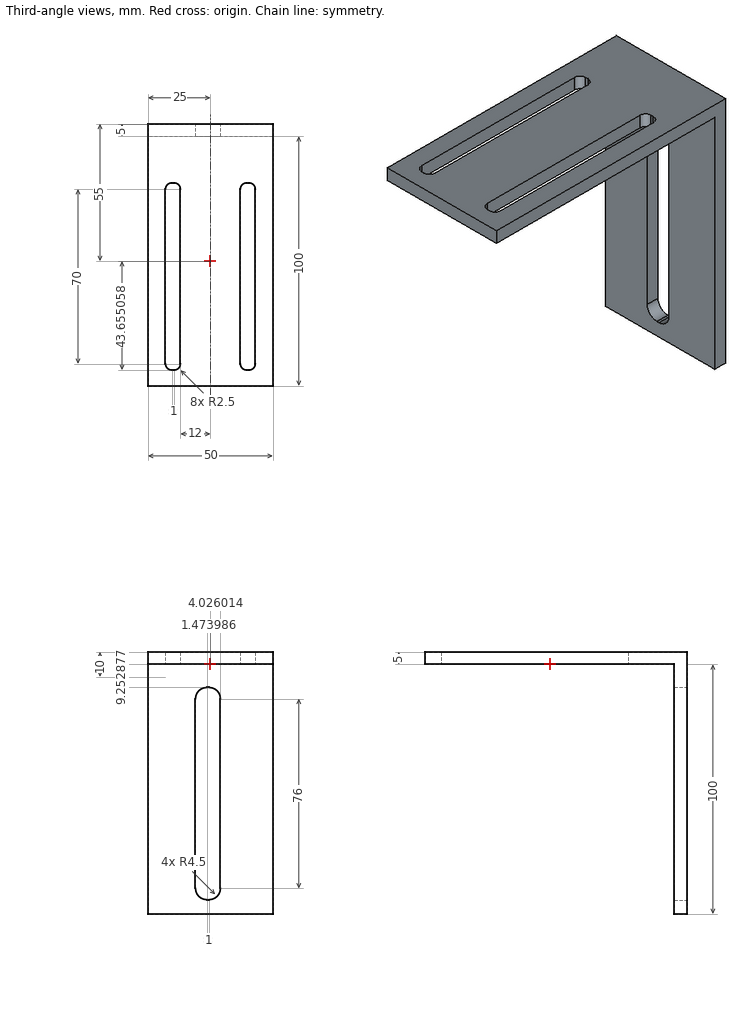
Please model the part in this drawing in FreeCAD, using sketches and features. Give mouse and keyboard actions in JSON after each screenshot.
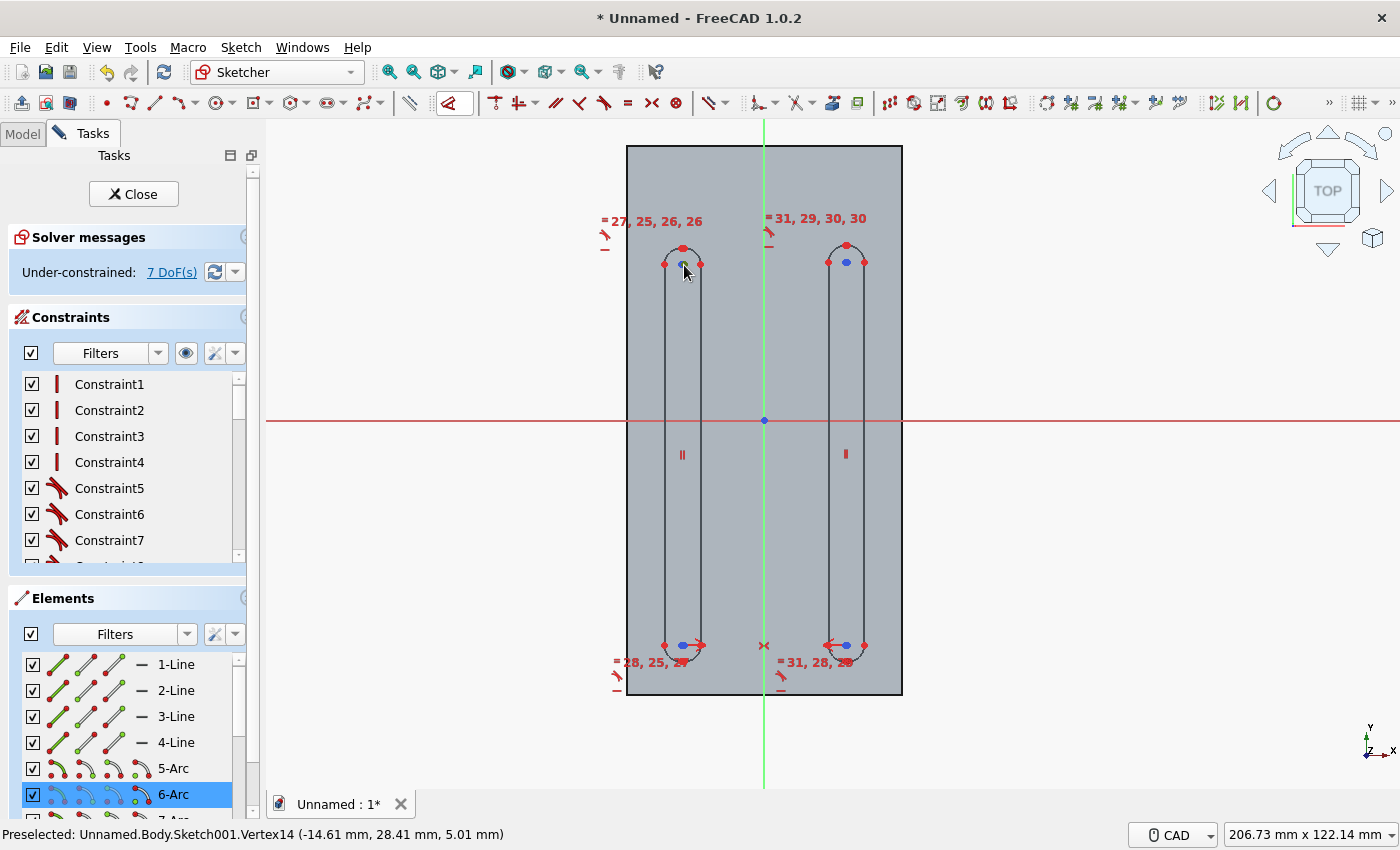
{"action": "scroll", "coordinate": [845, 262], "scroll_direction": "up", "scroll_amount": 8}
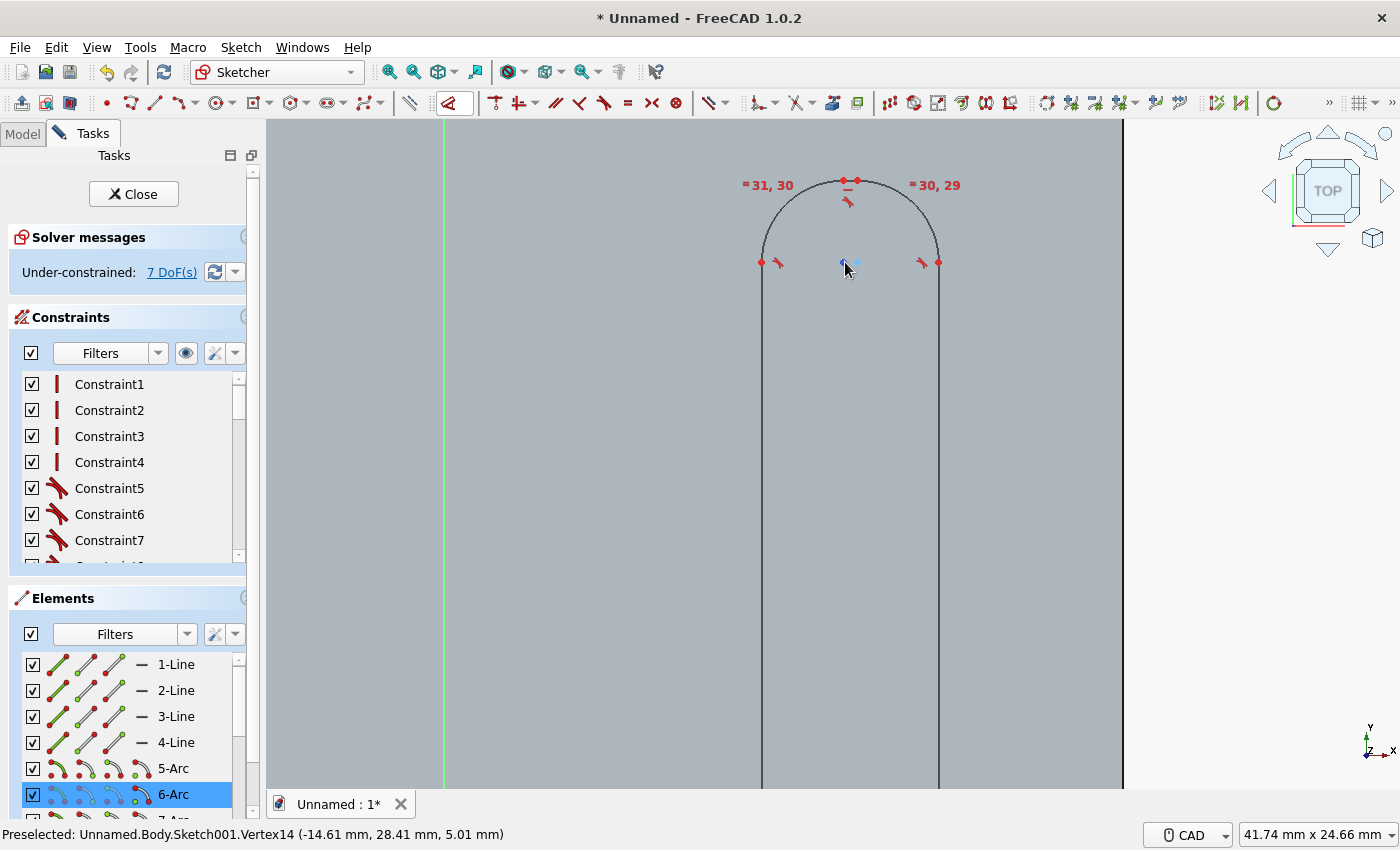
{"action": "left_click", "coordinate": [844, 262]}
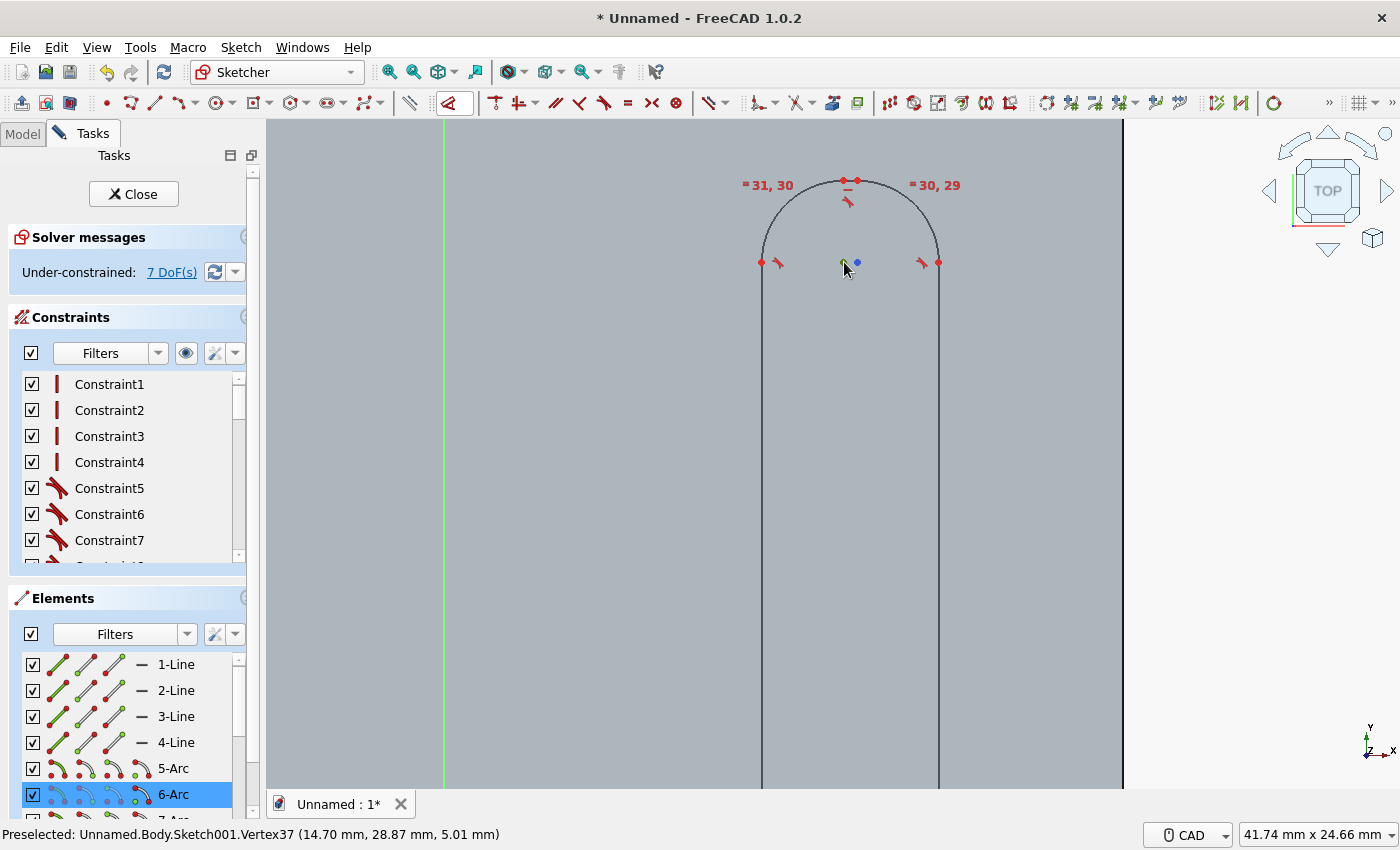
{"action": "left_click", "coordinate": [444, 717]}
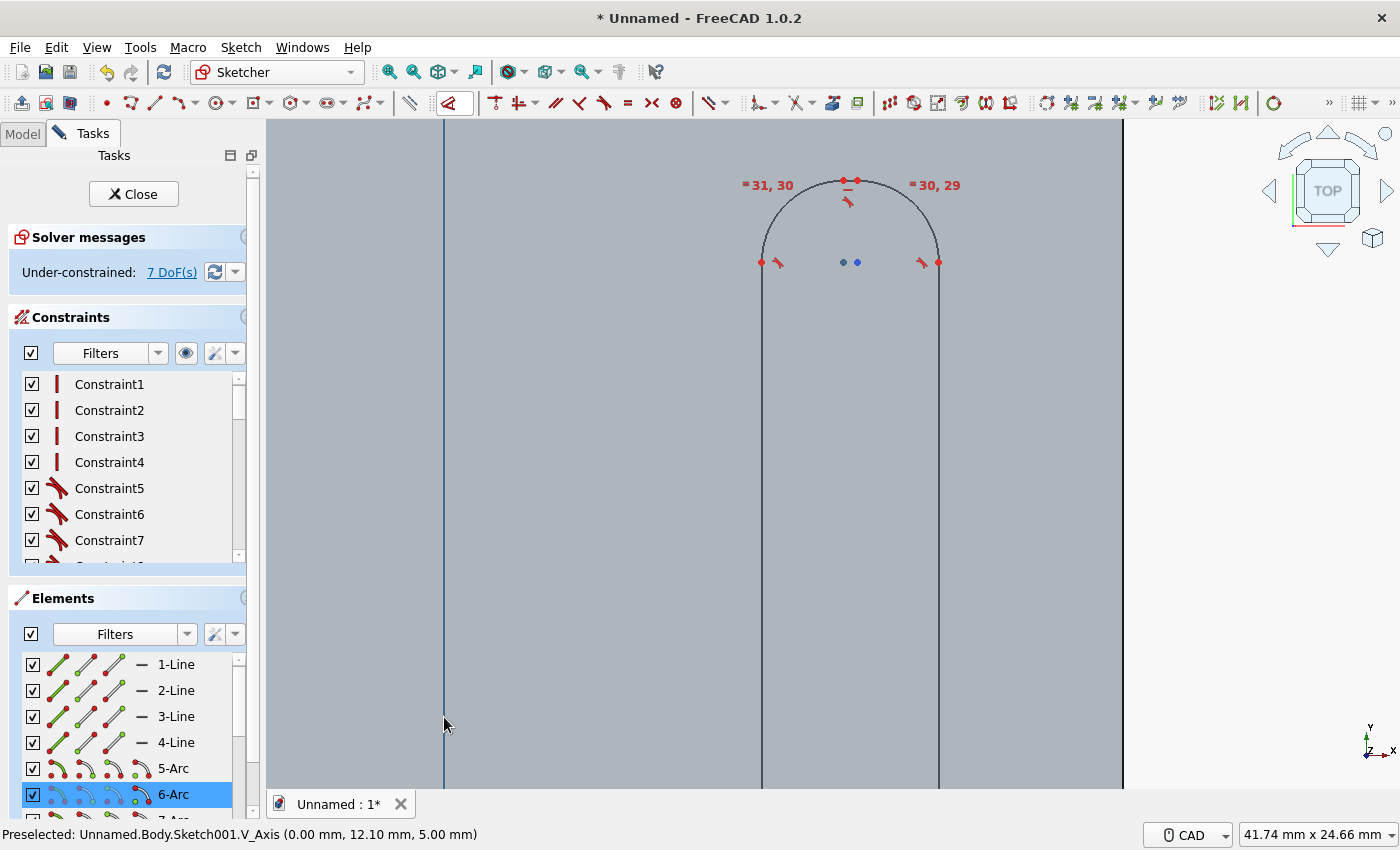
{"action": "key", "text": "s"}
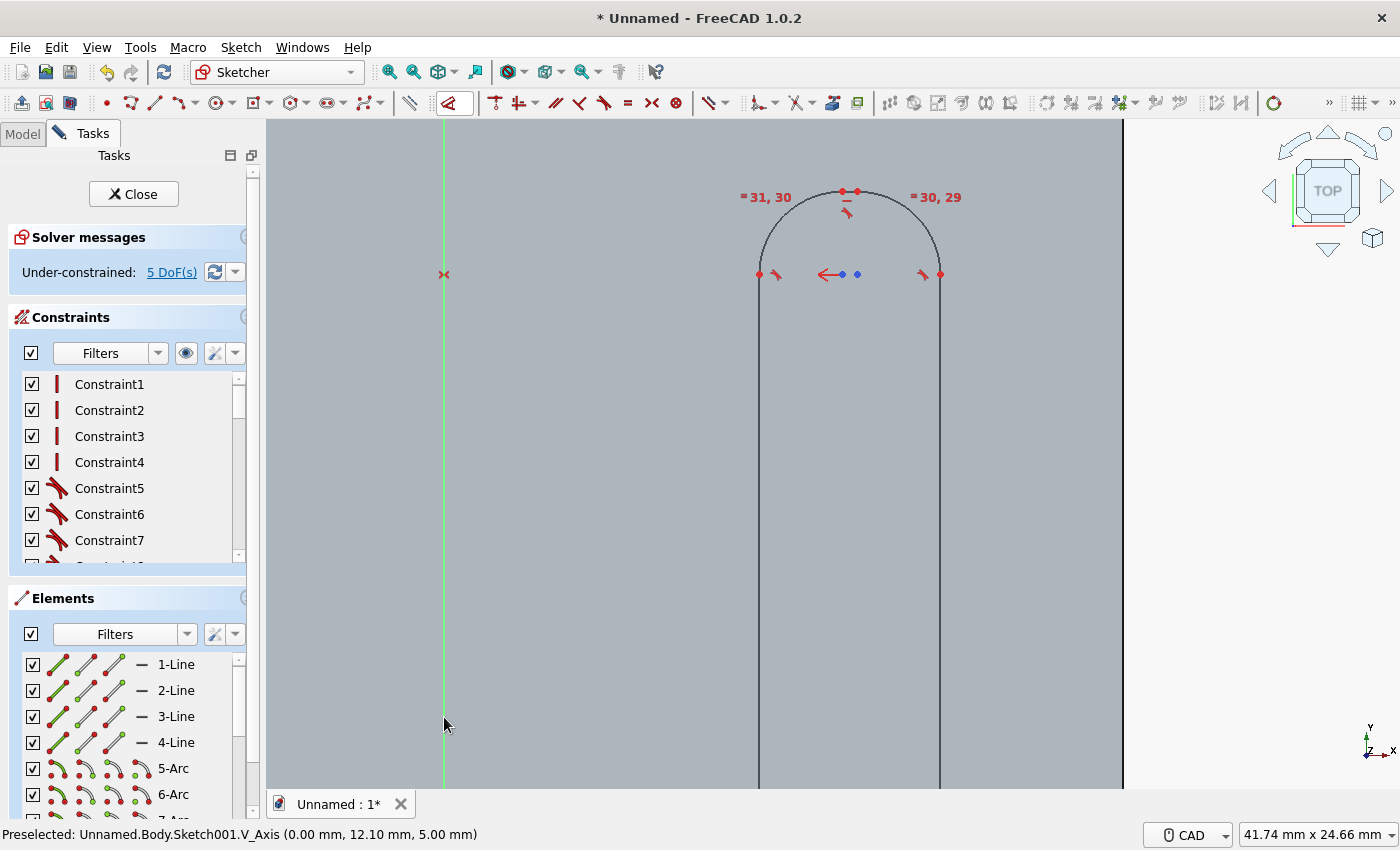
{"action": "scroll", "coordinate": [846, 262], "scroll_direction": "down", "scroll_amount": 8}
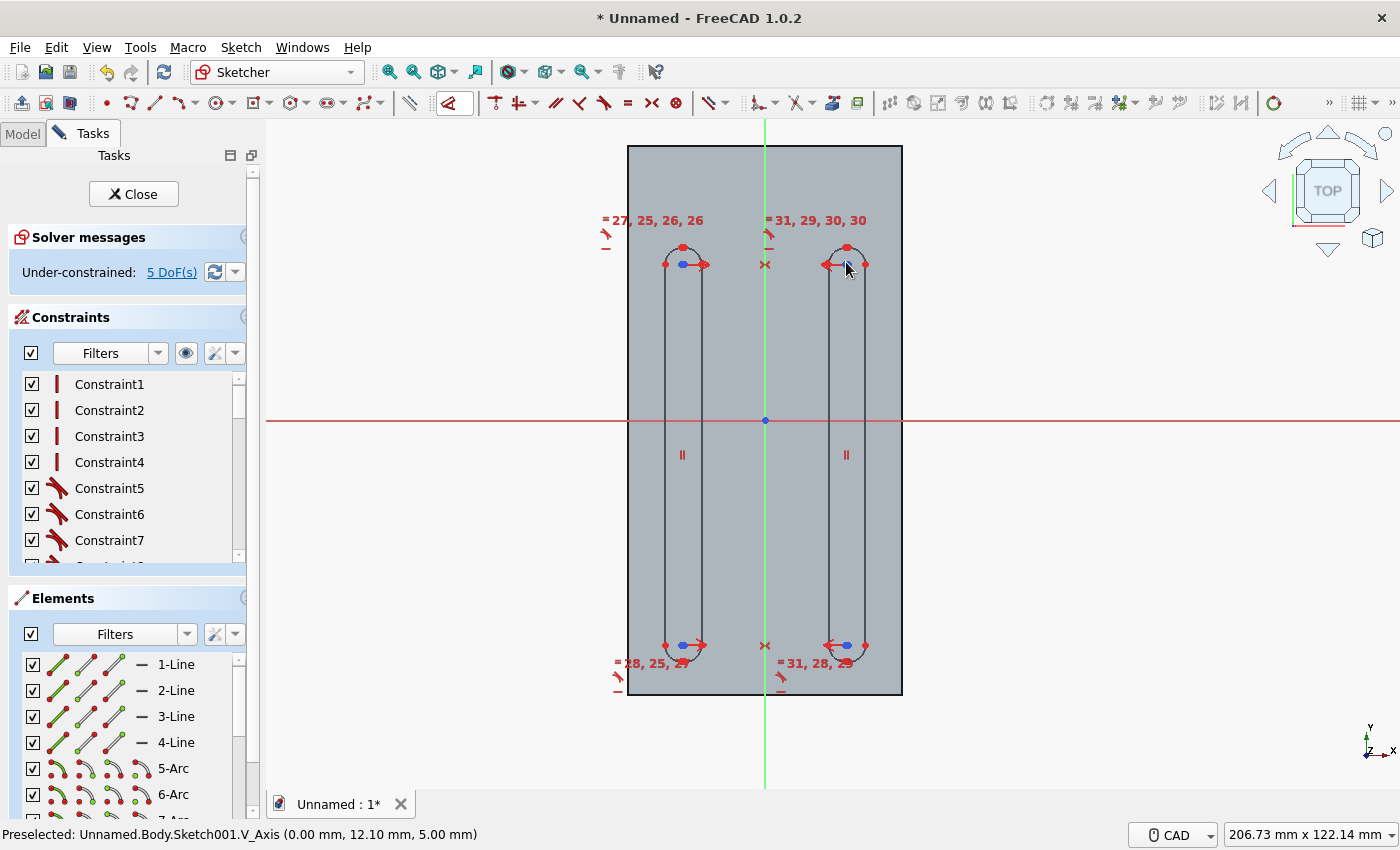
{"action": "scroll", "coordinate": [692, 660], "scroll_direction": "up", "scroll_amount": 6}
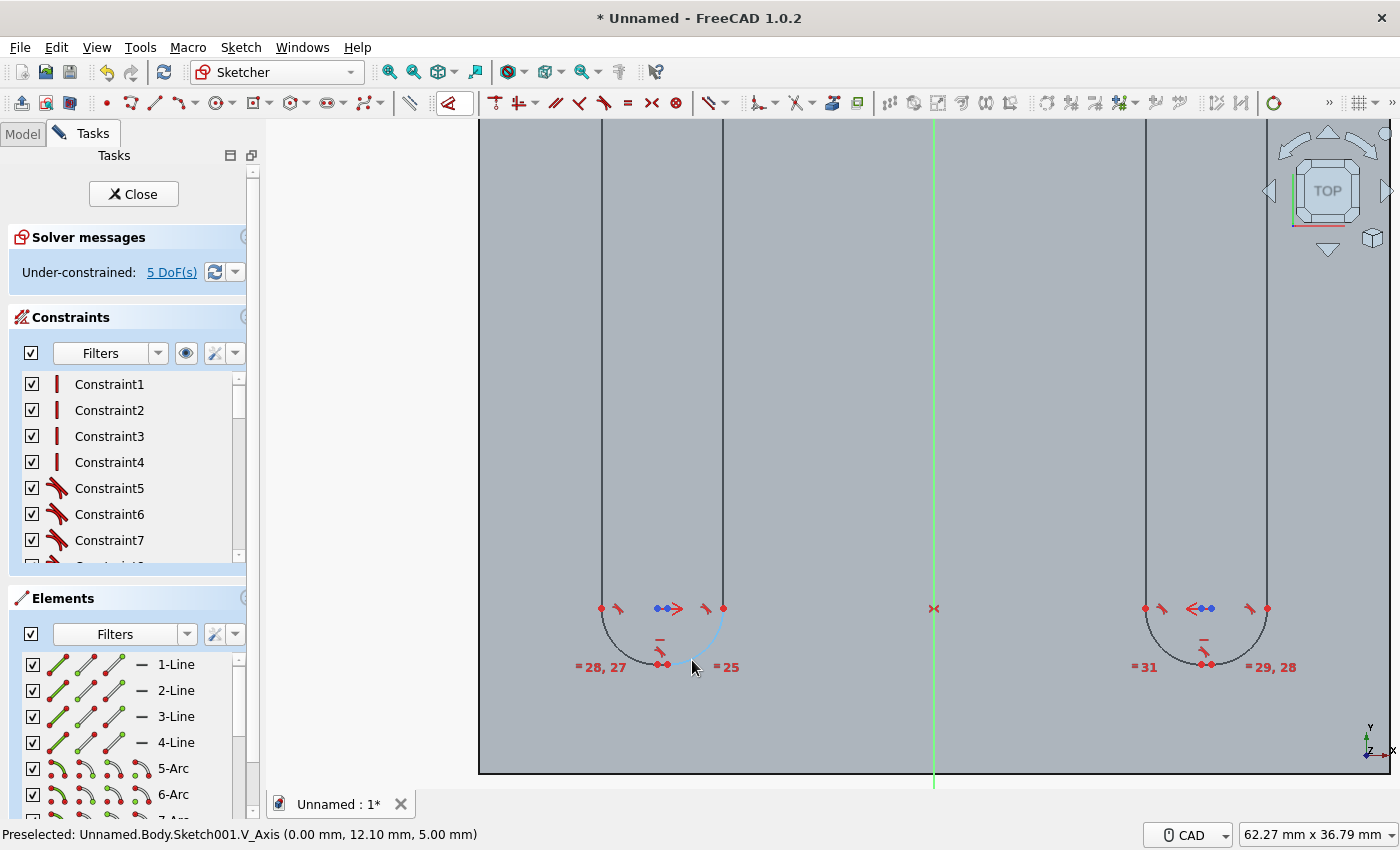
{"action": "left_click", "coordinate": [693, 659]}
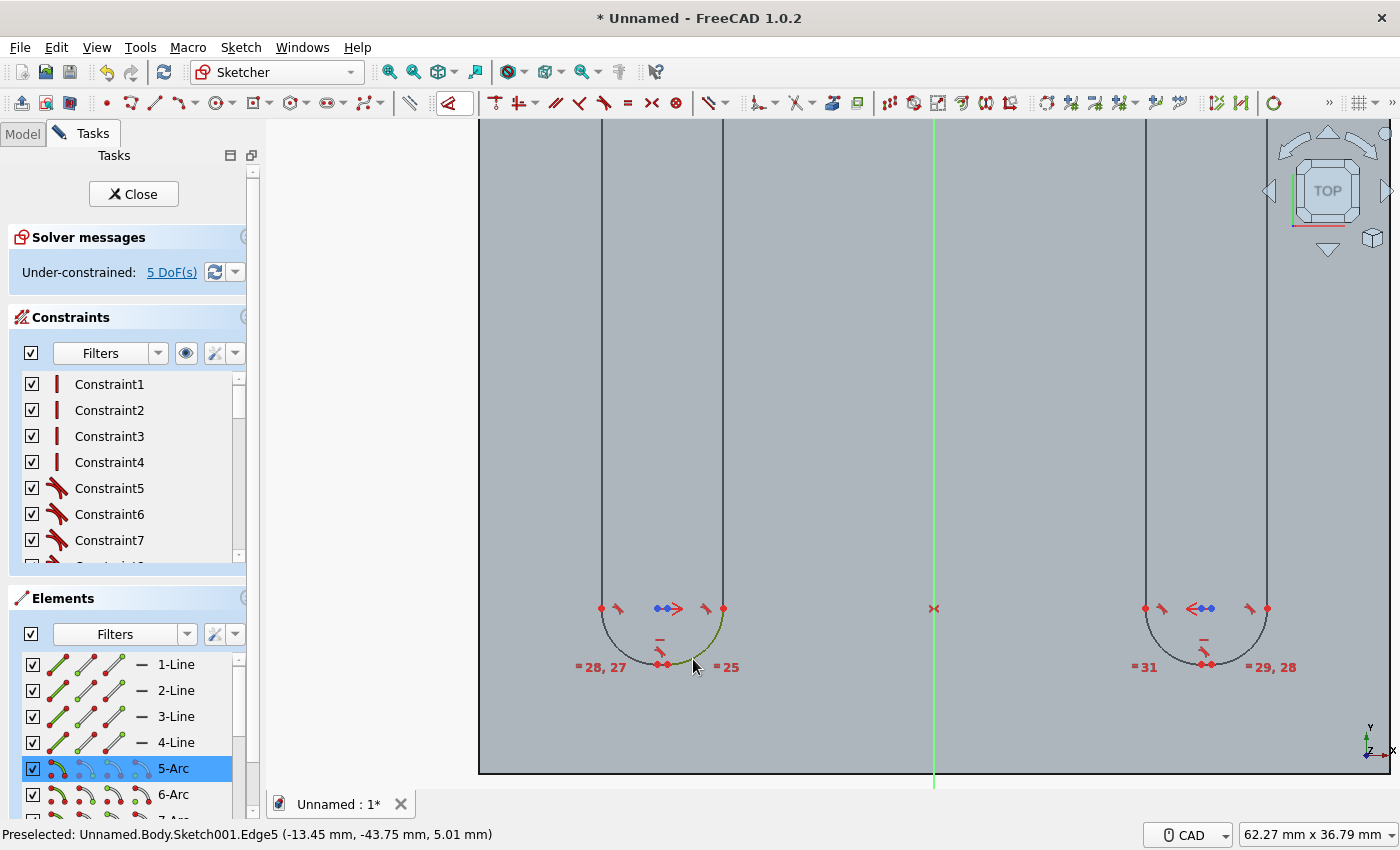
{"action": "key", "text": "k r"}